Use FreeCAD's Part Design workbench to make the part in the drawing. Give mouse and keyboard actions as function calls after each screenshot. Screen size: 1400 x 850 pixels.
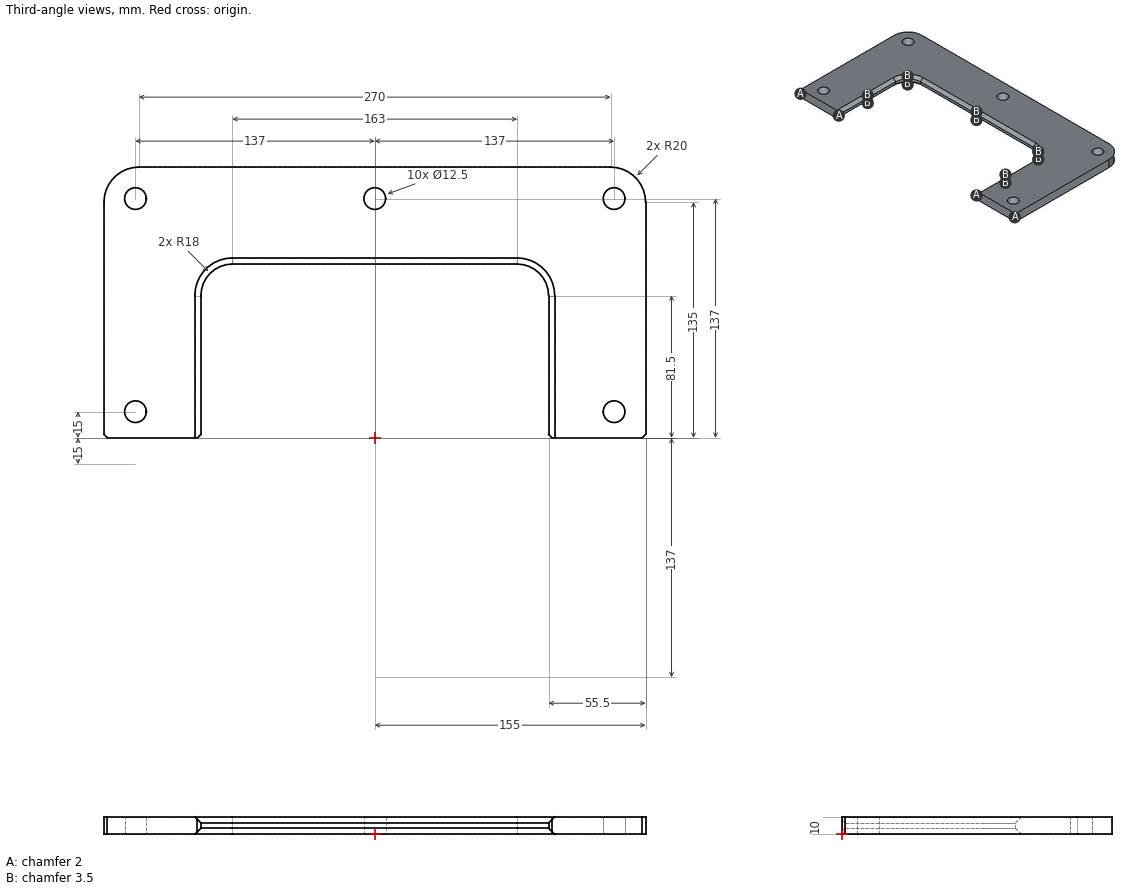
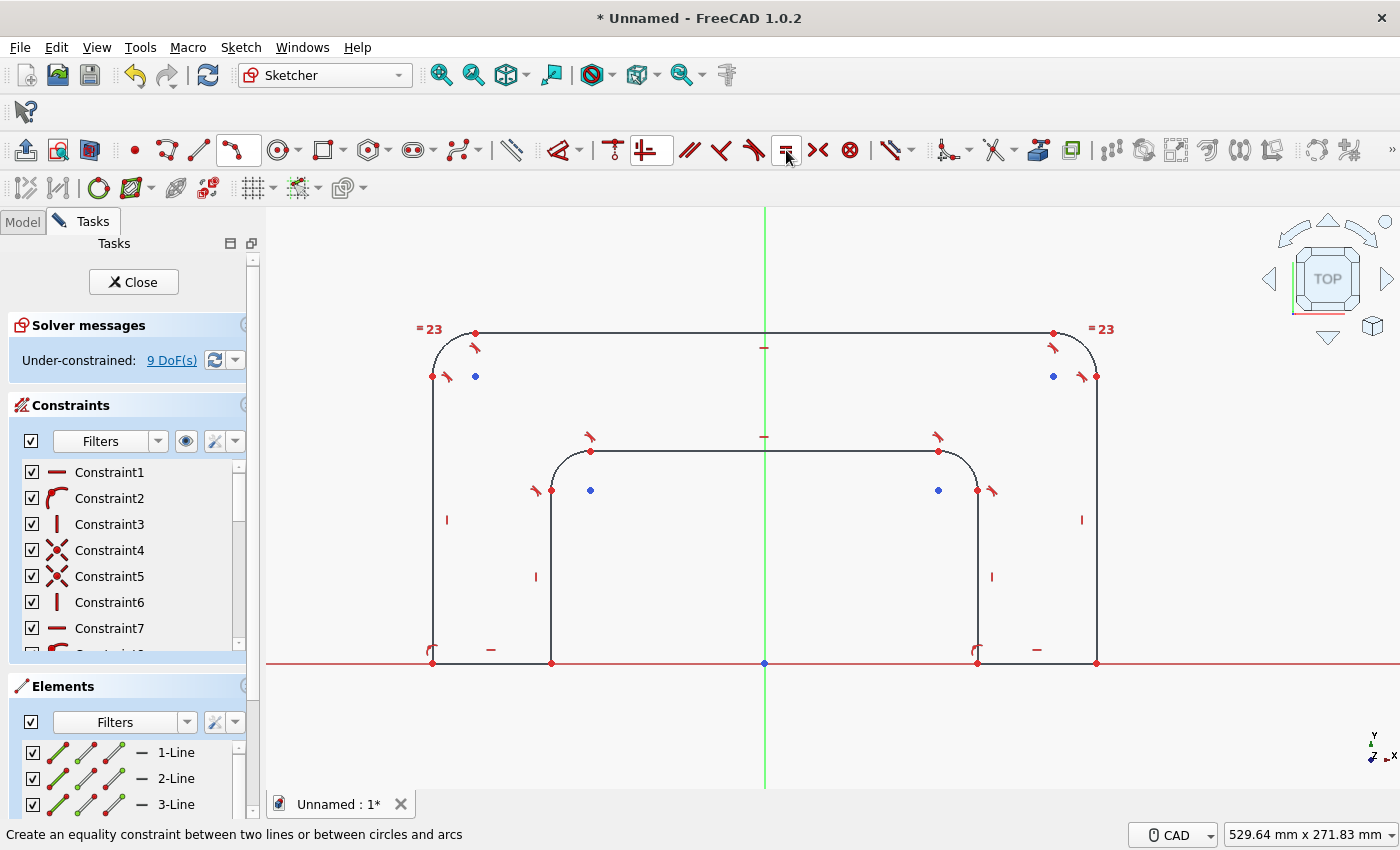
click(973, 472)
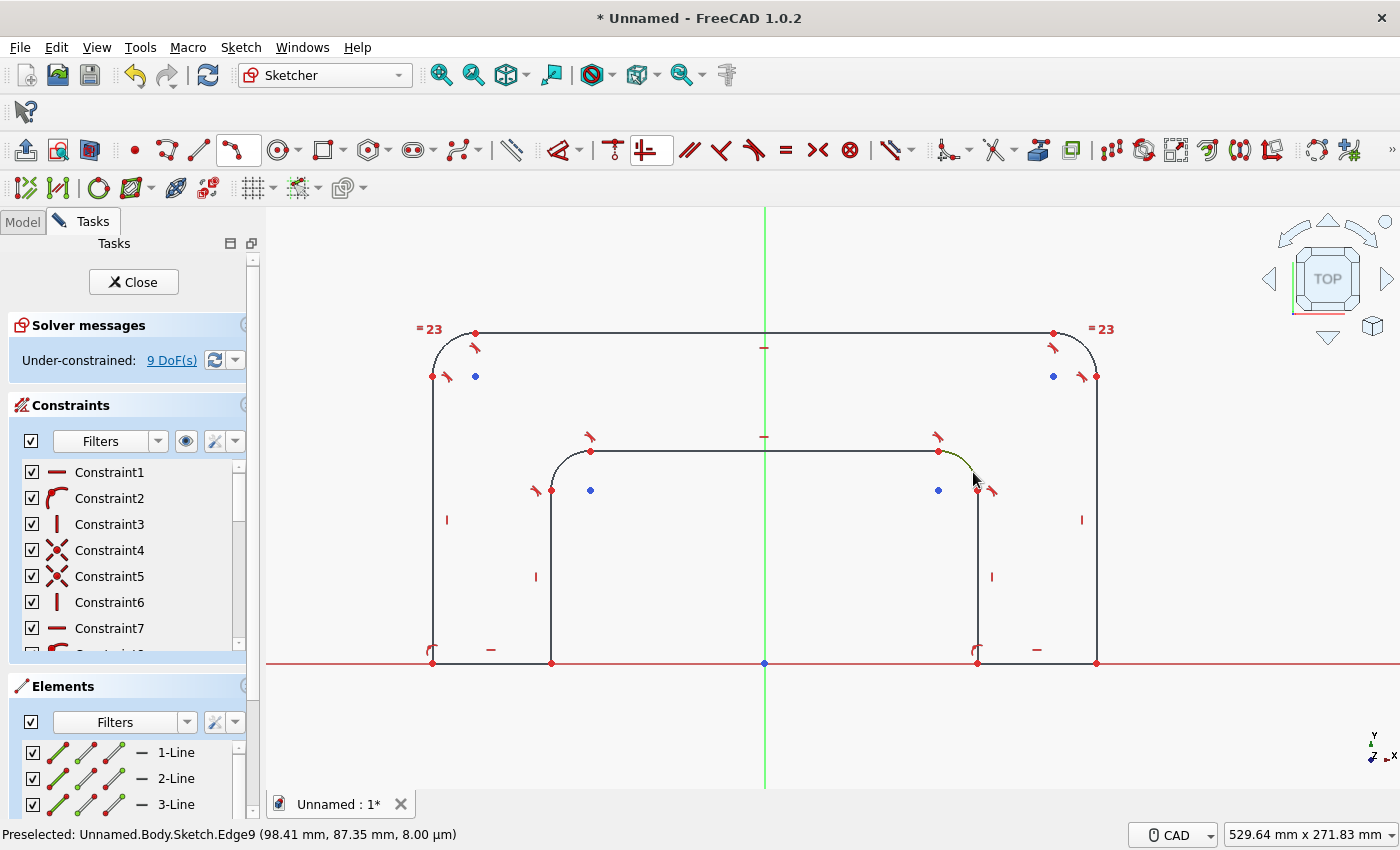
click(572, 455)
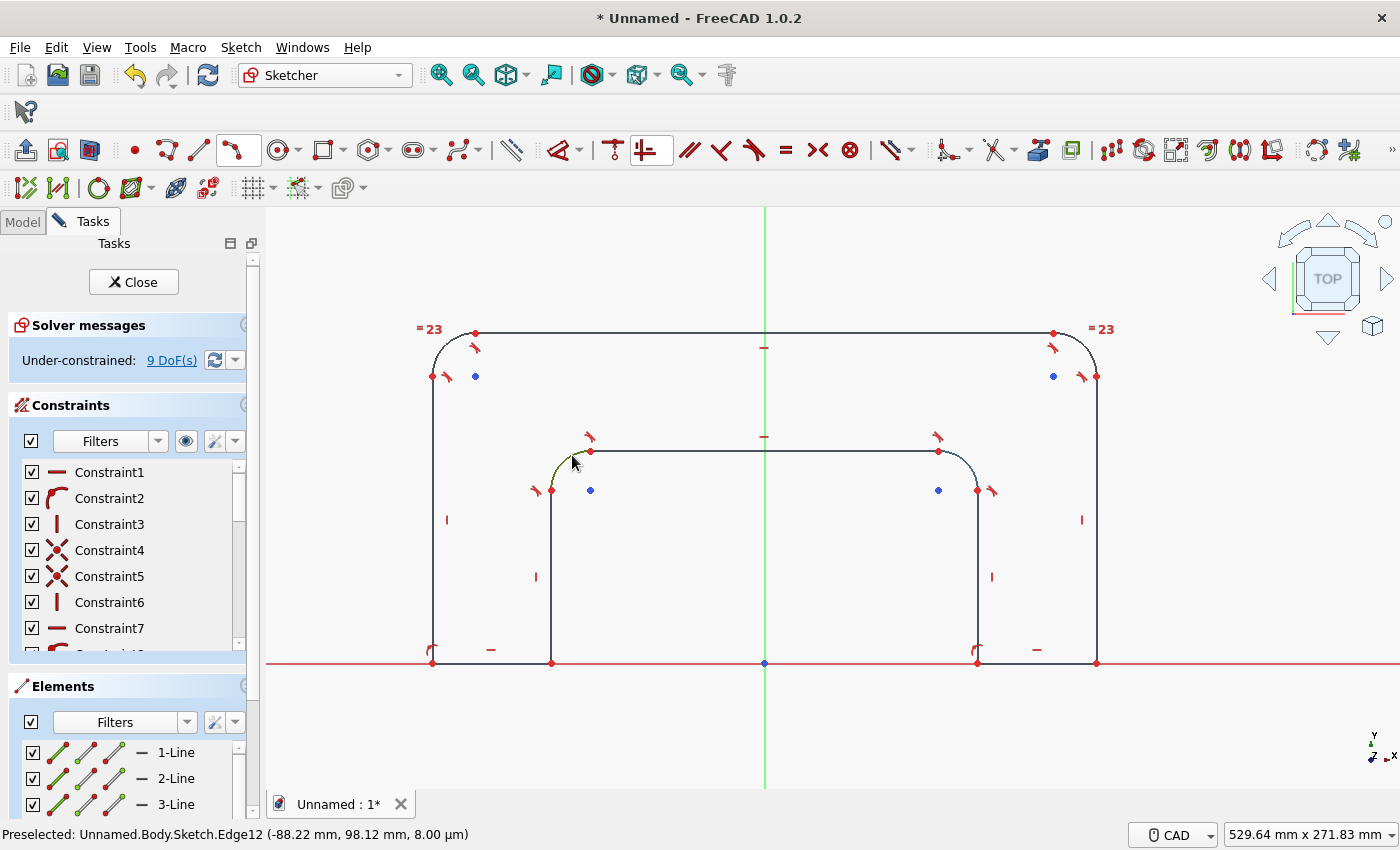
key(e)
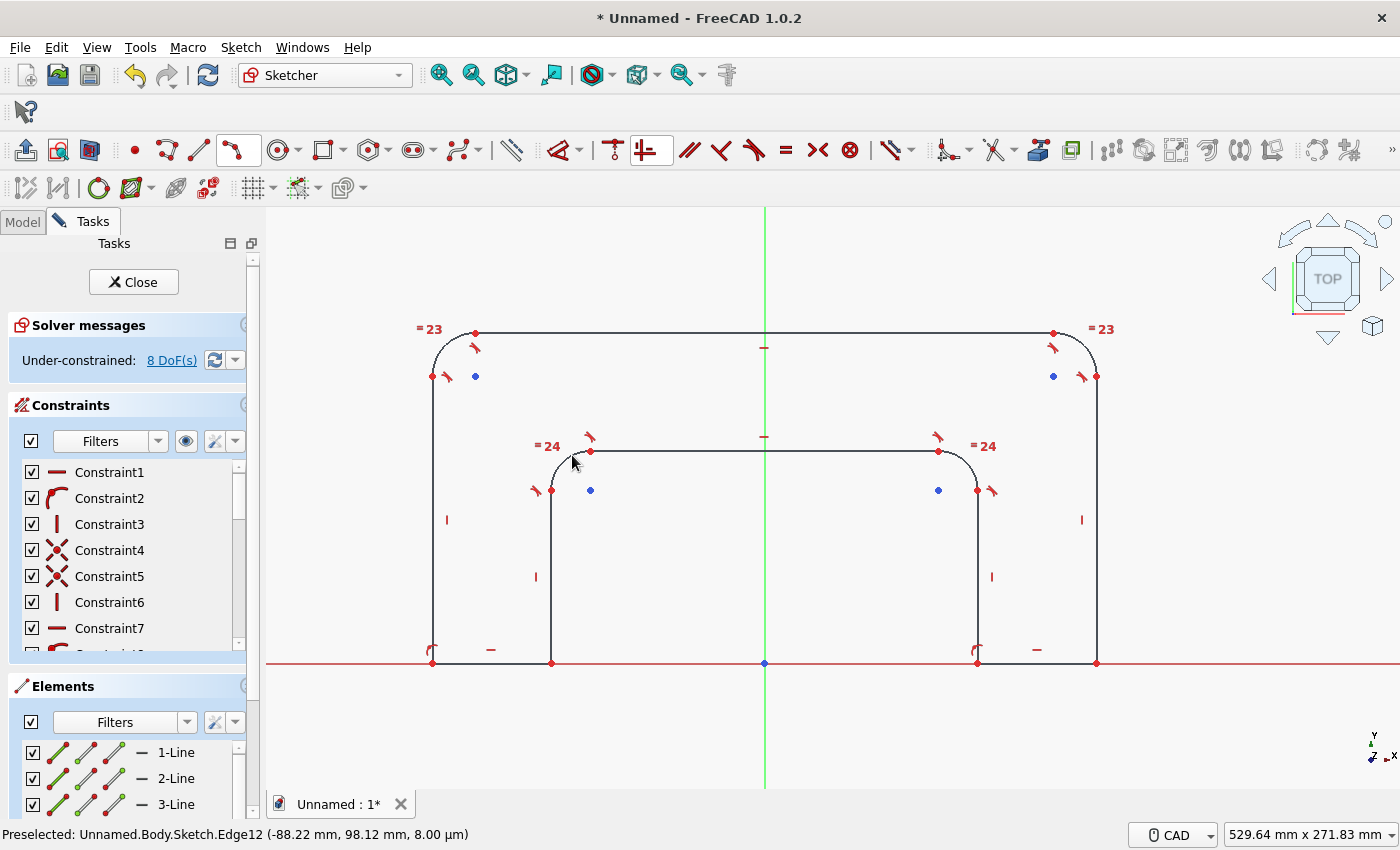
click(973, 472)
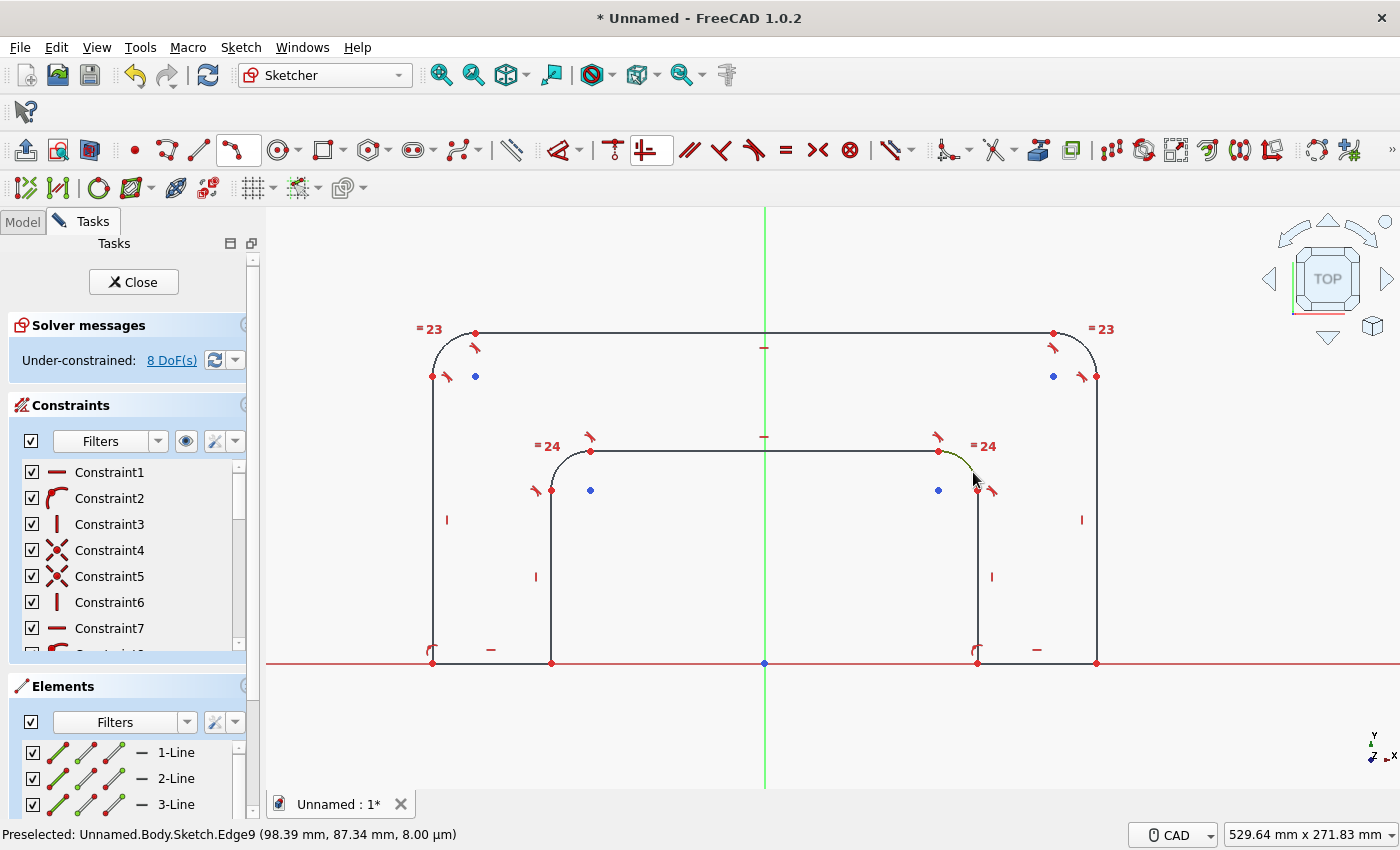
key(k)
key(r)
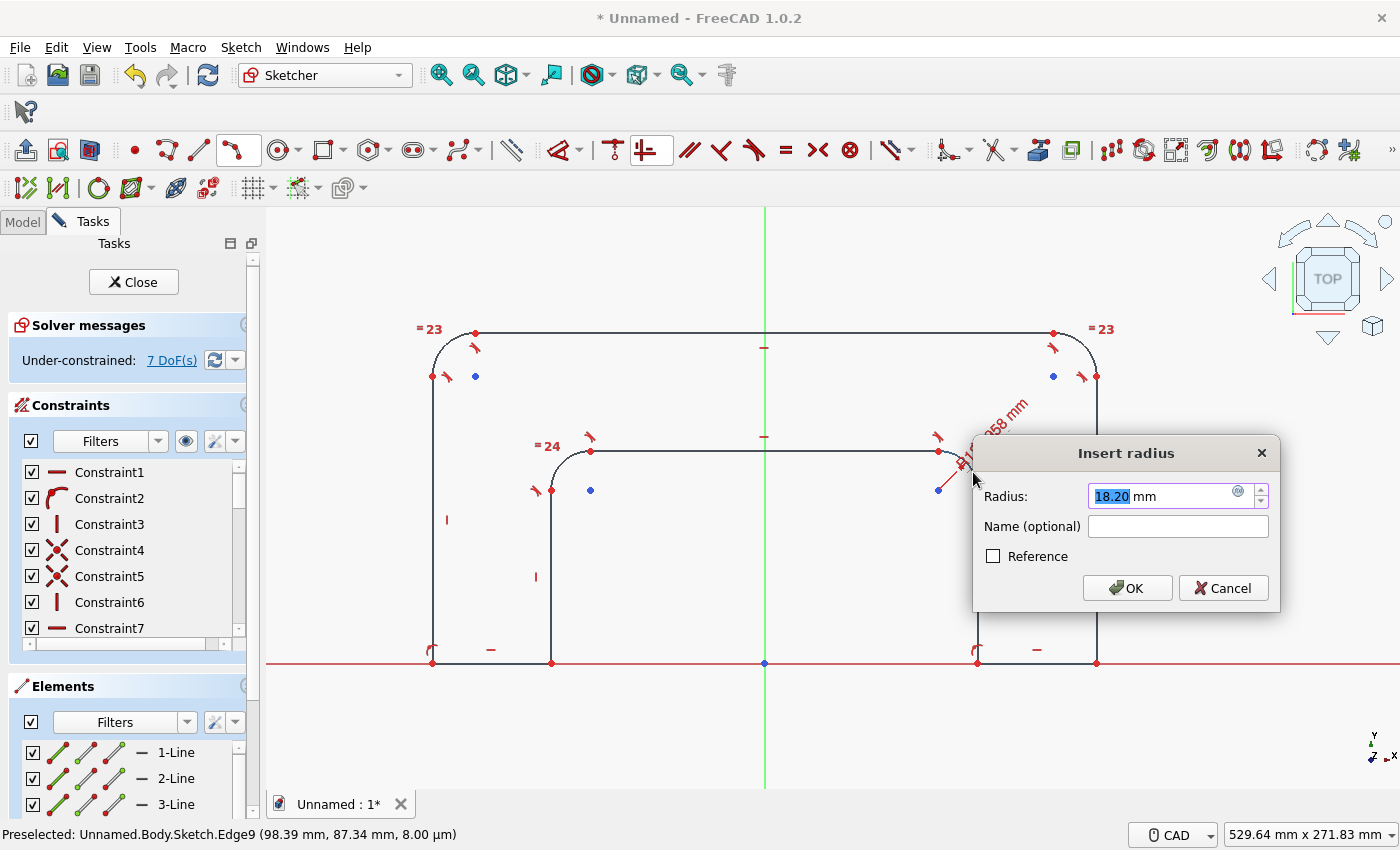
text(18)
key(Return)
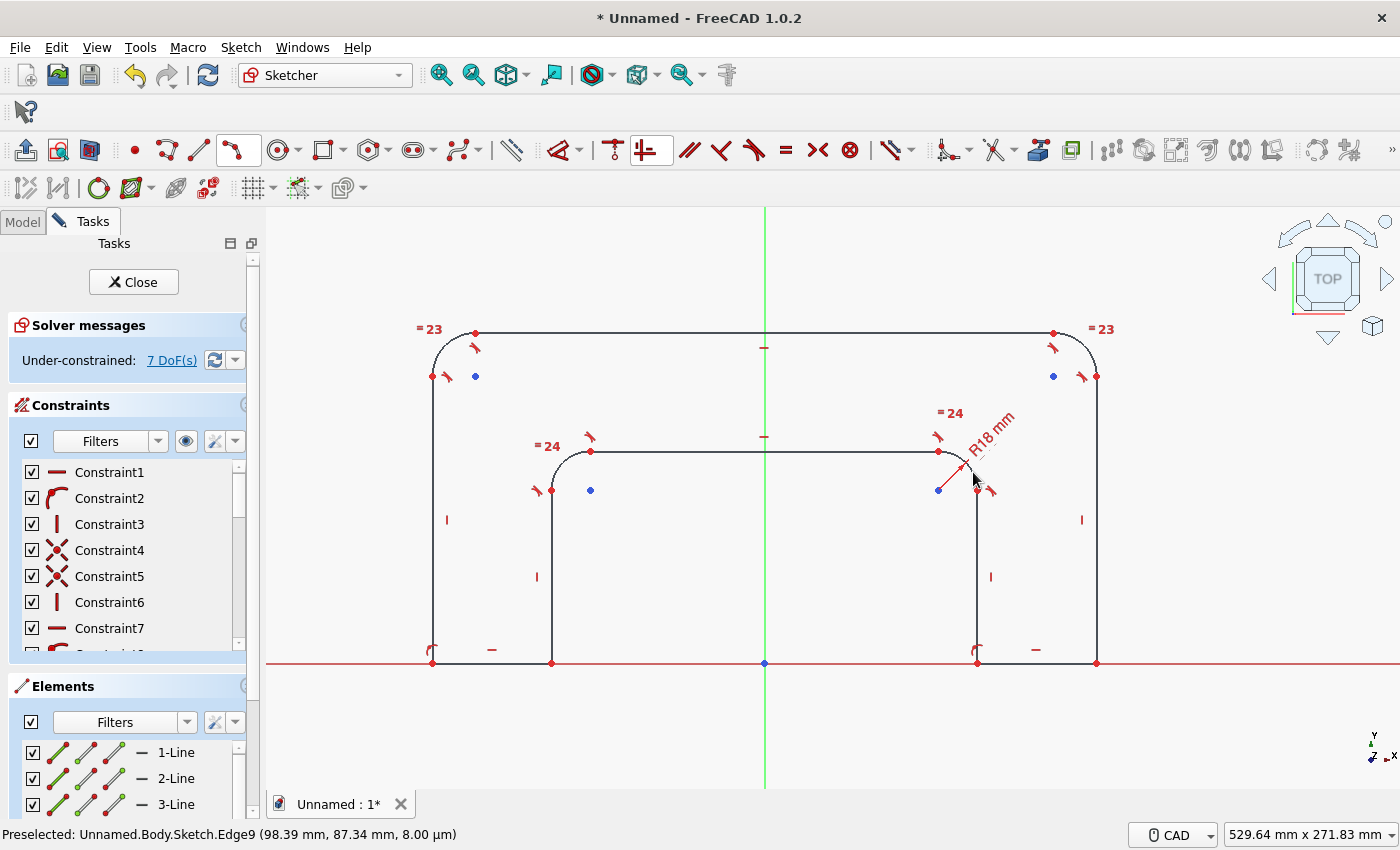
click(1092, 356)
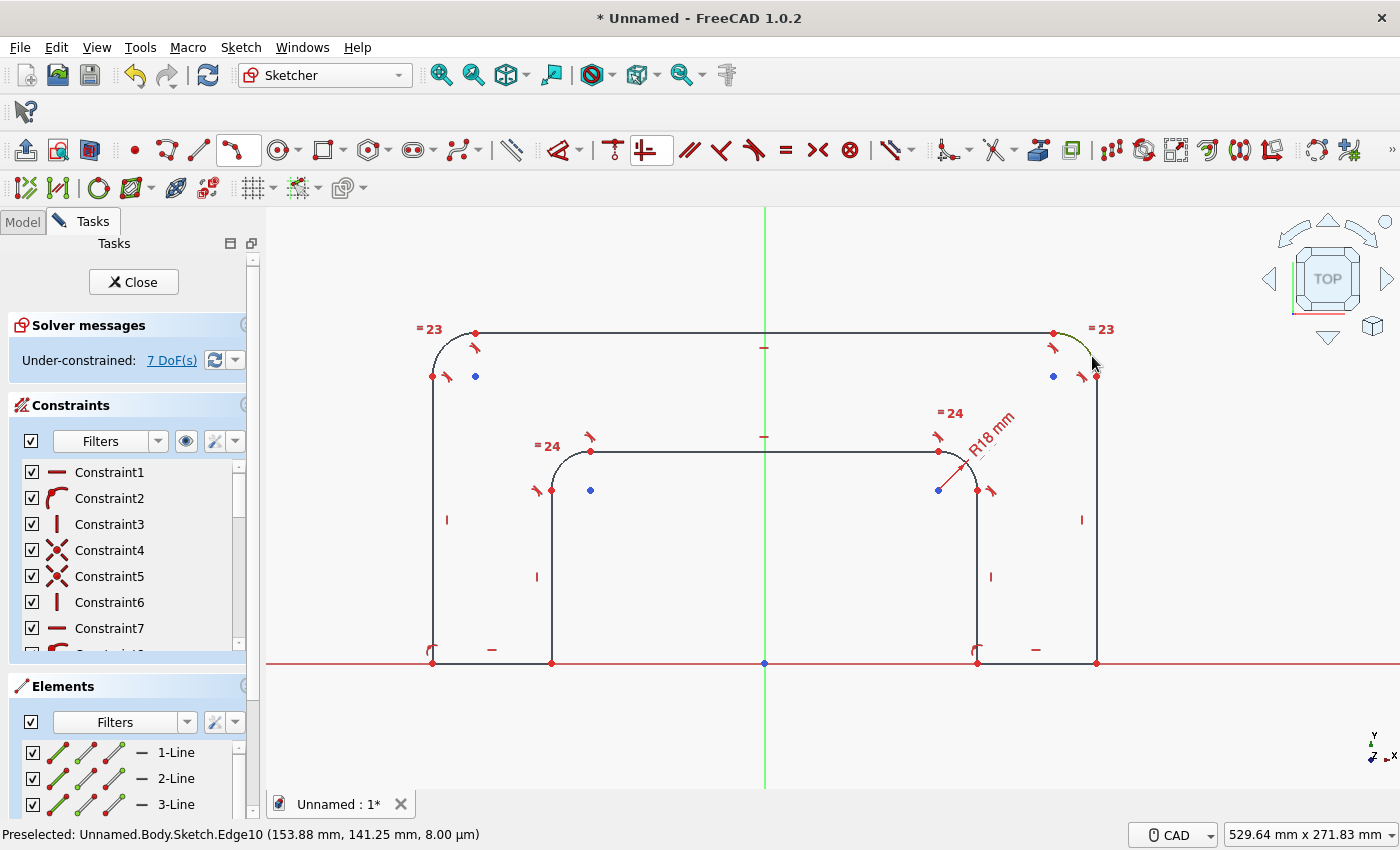
key(k)
key(r)